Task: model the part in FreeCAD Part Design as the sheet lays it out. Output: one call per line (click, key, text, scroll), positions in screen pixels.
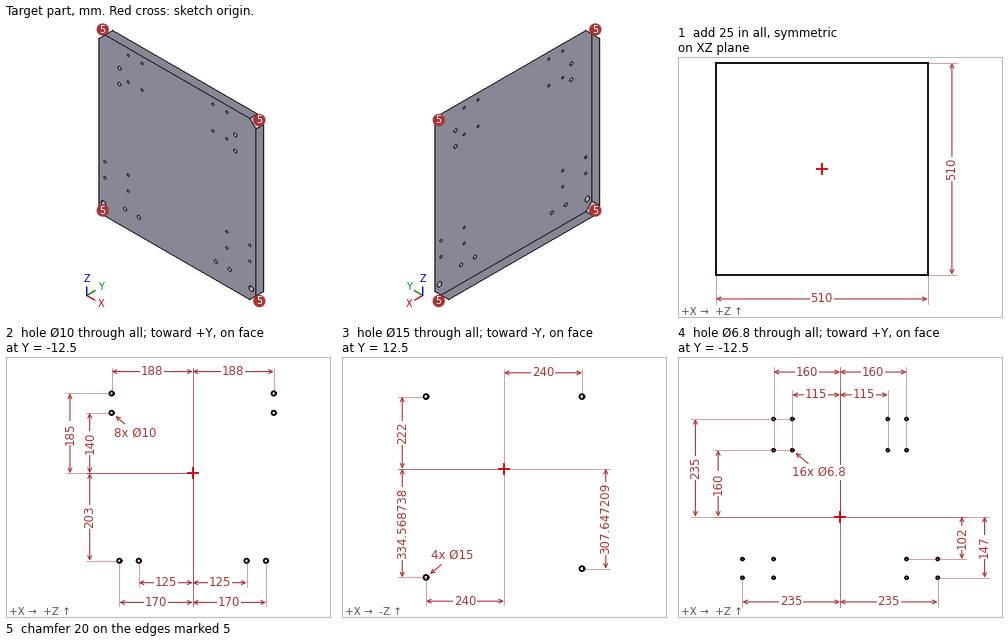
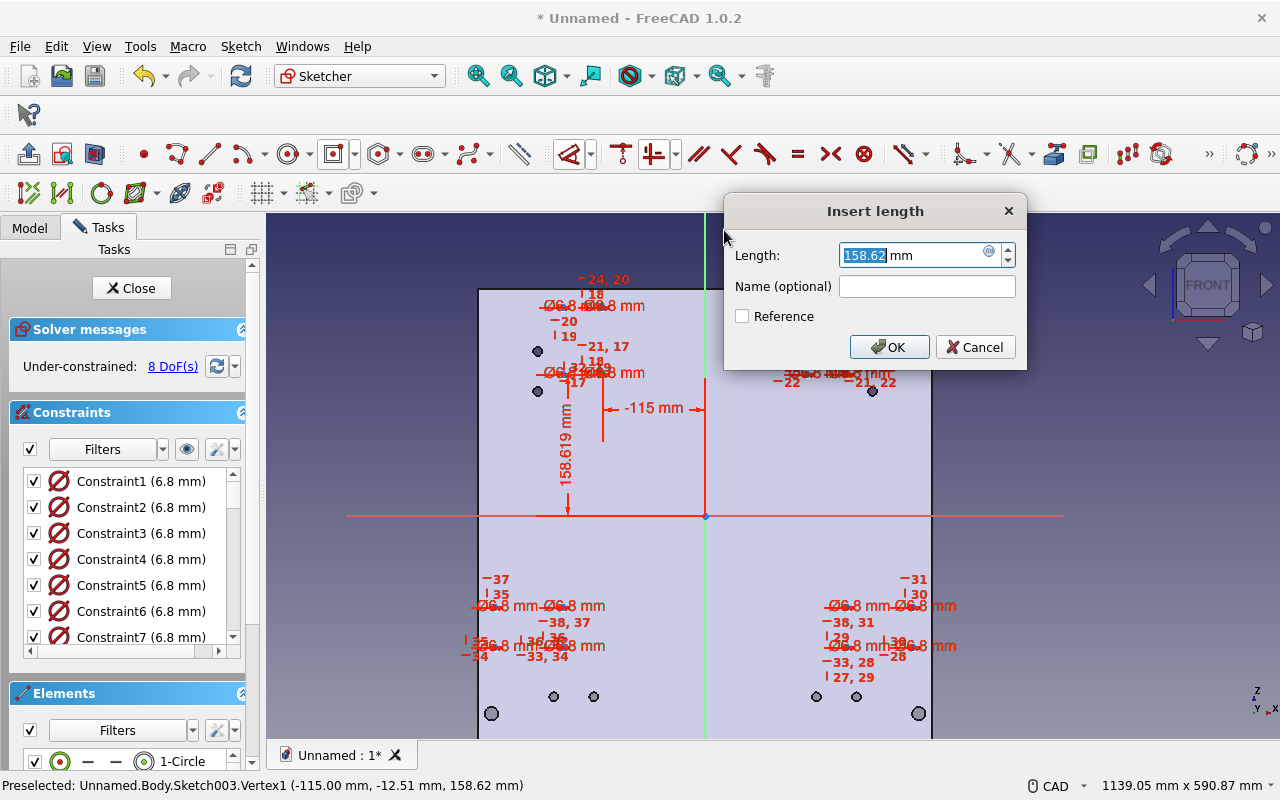
text(160)
key(Return)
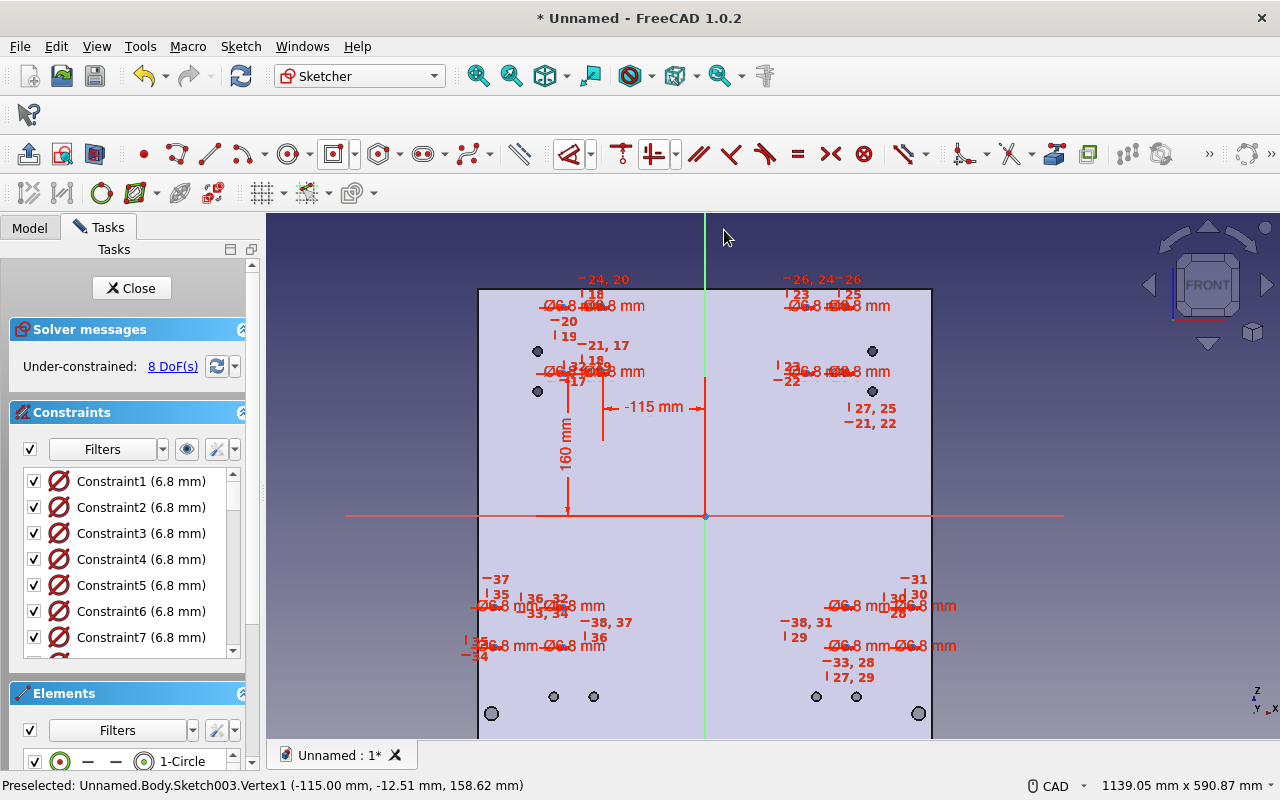
click(563, 374)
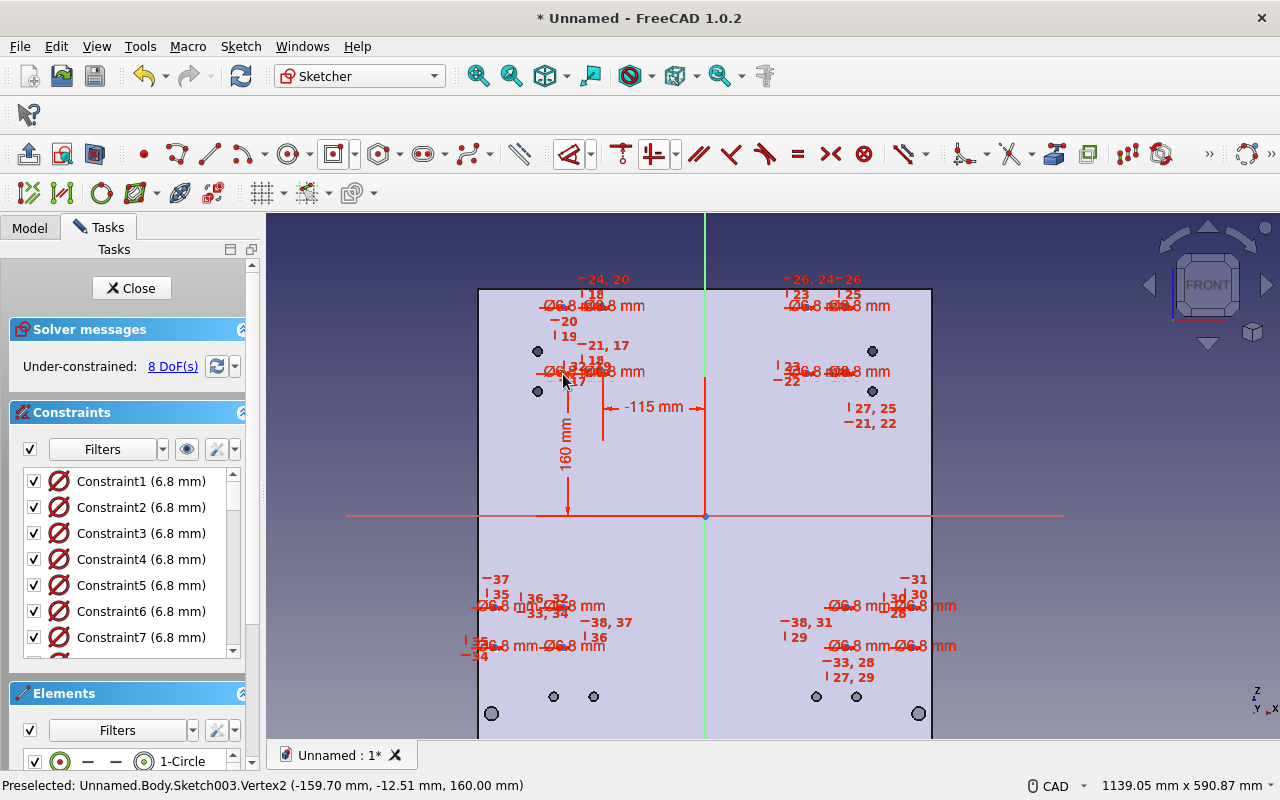
click(590, 154)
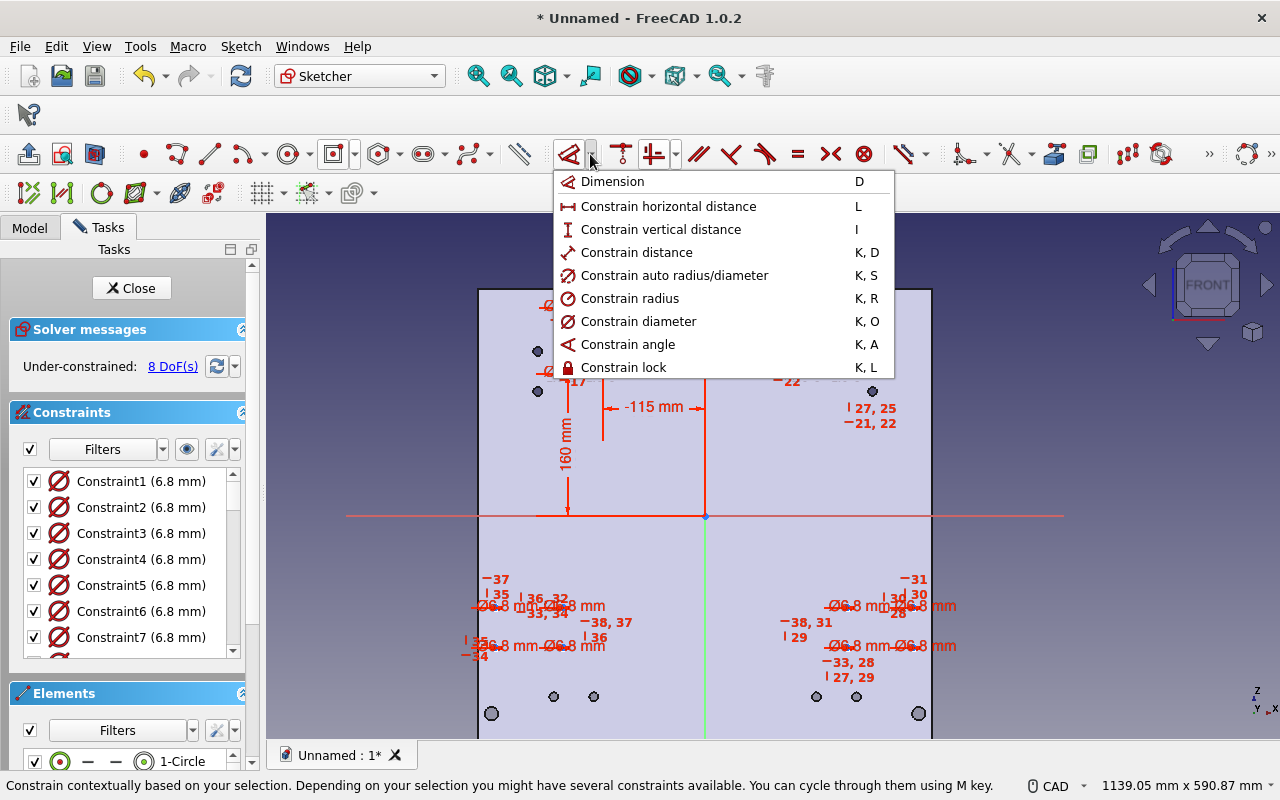
click(724, 206)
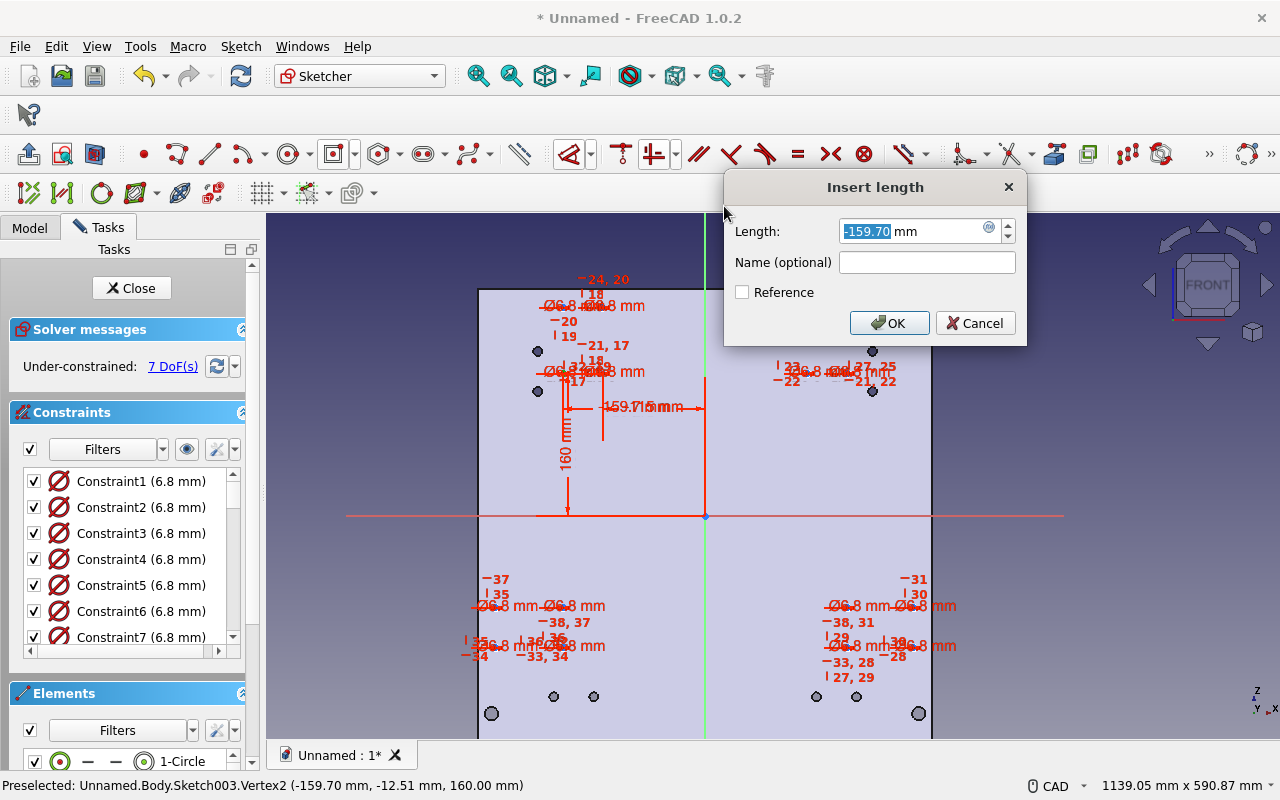
text(-160)
key(Return)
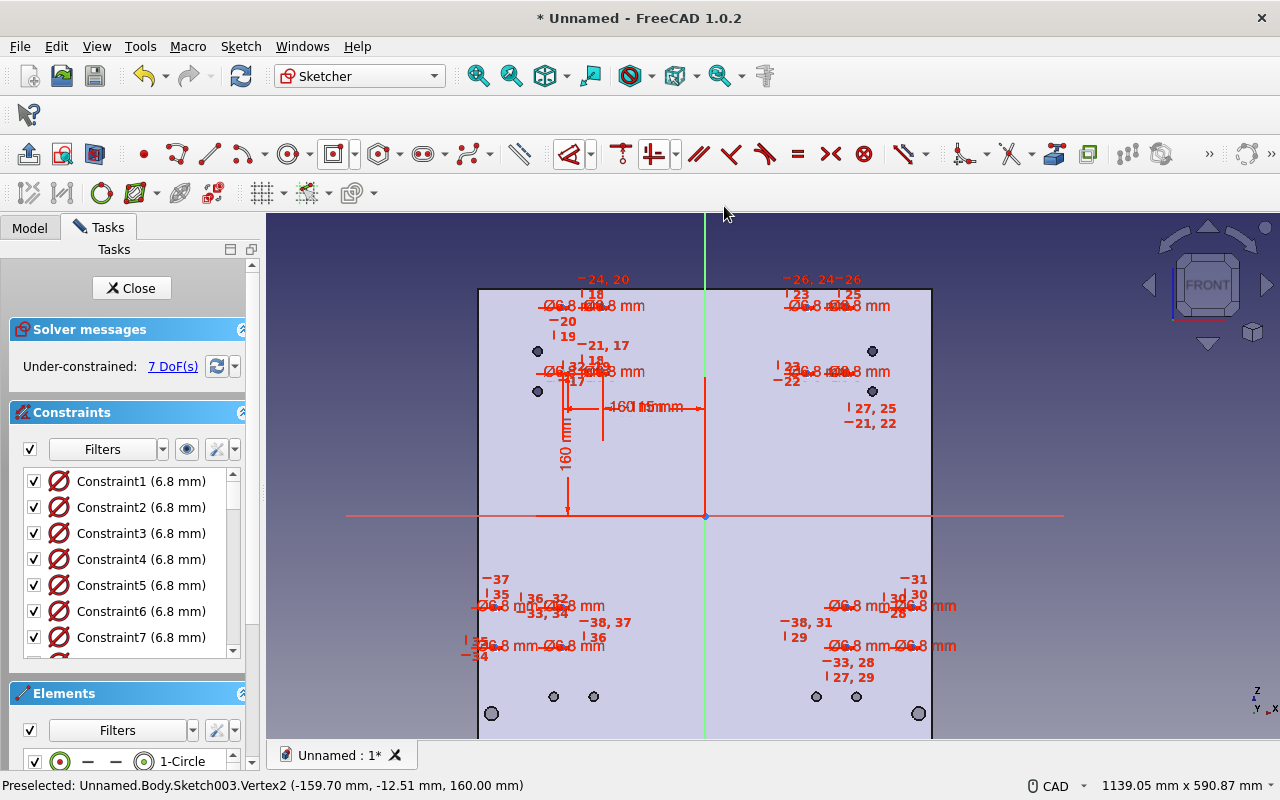
click(603, 308)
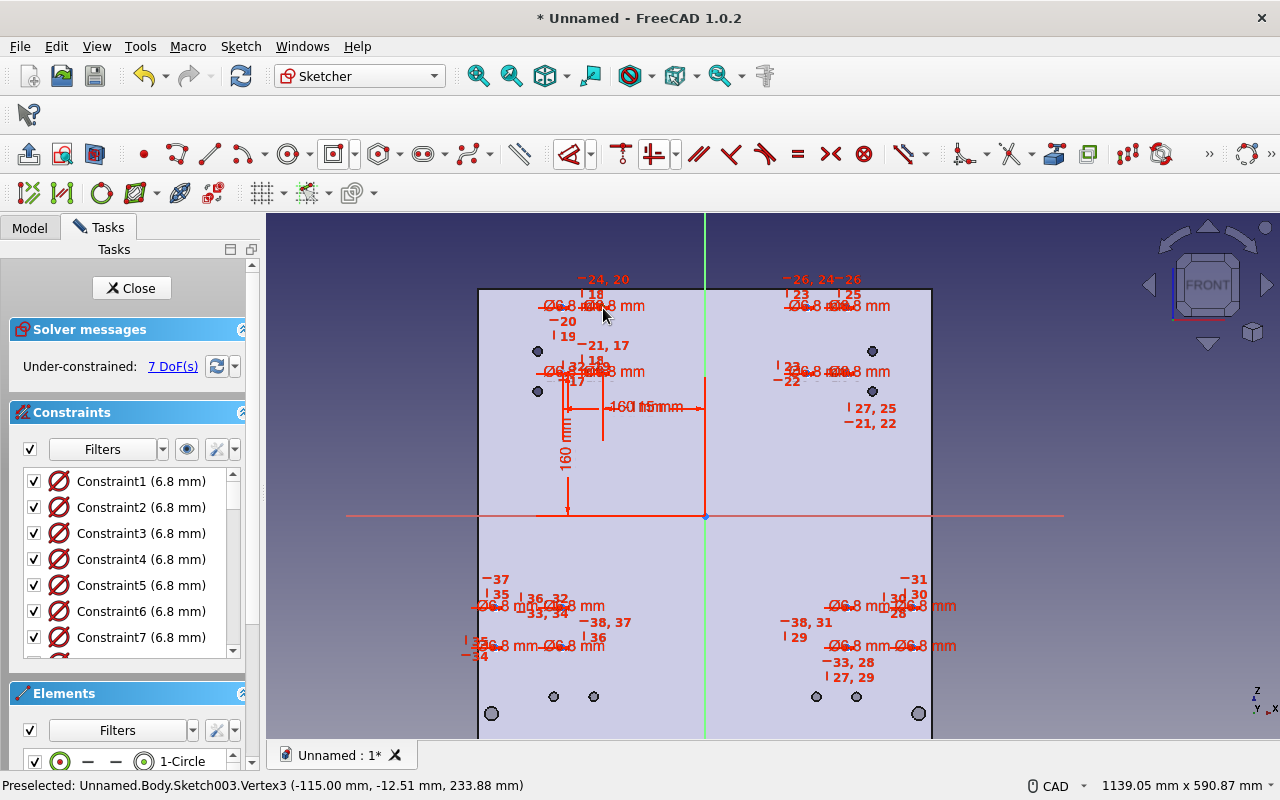
click(590, 154)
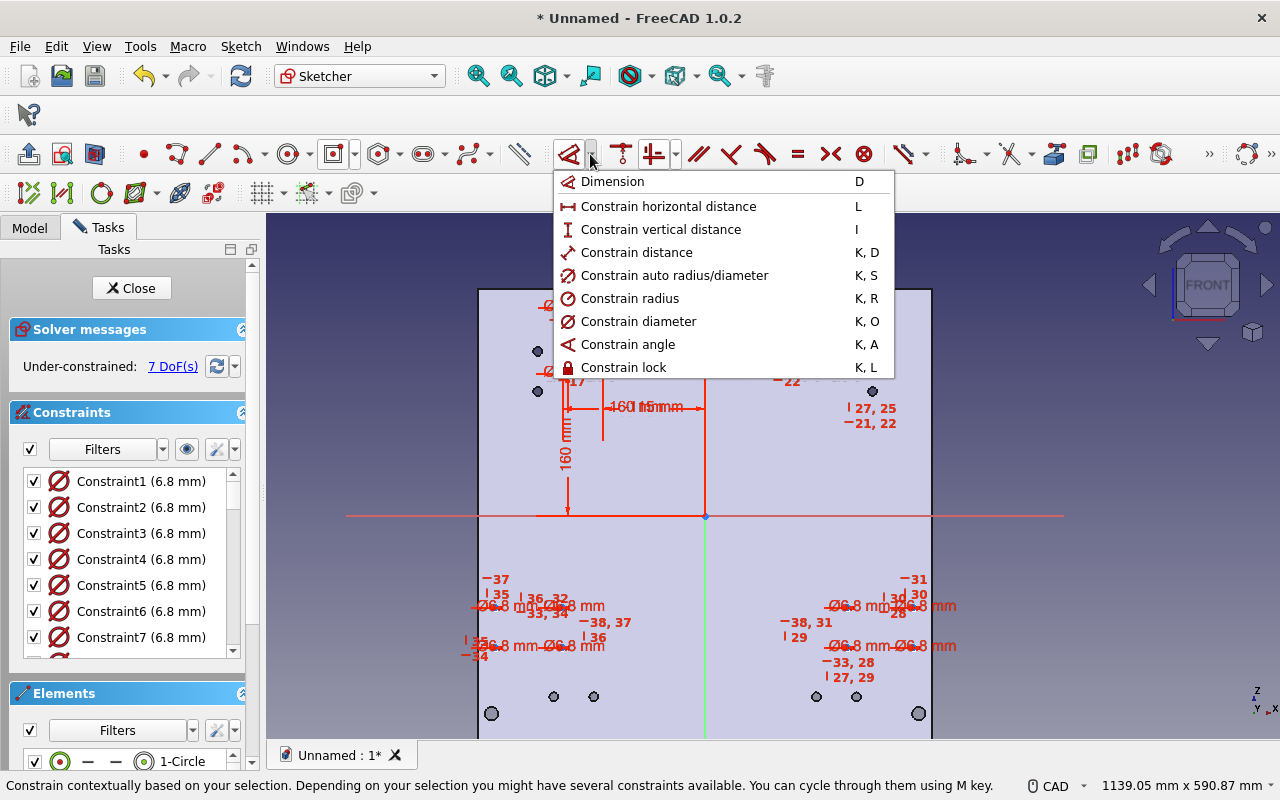
click(724, 230)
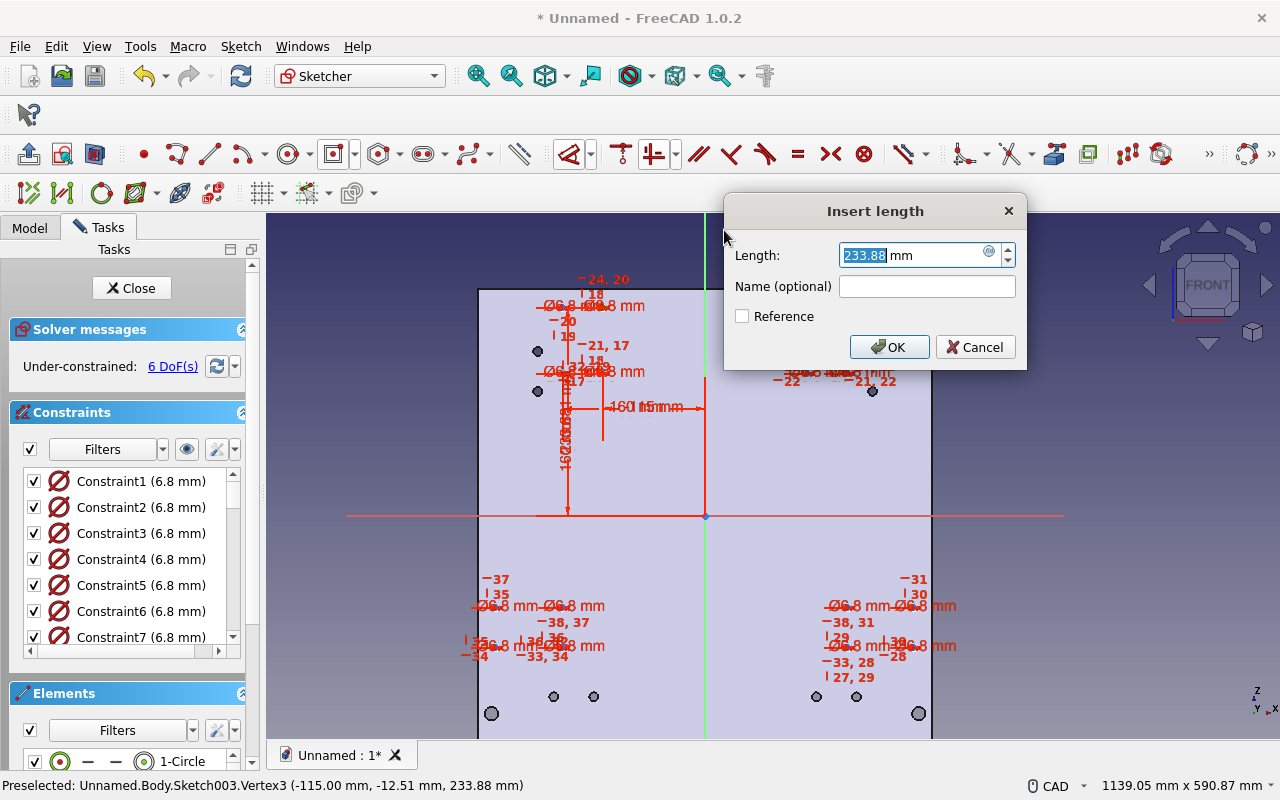
text(235)
key(Return)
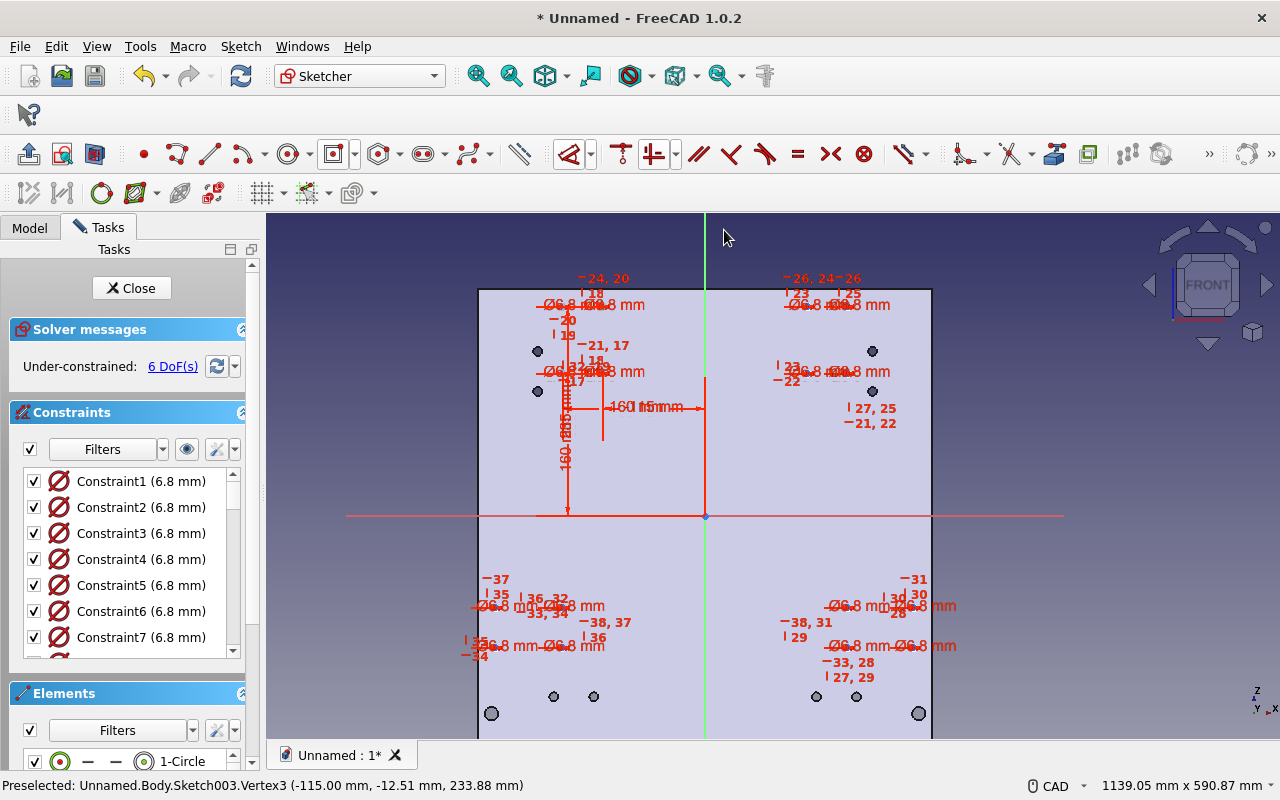
click(848, 374)